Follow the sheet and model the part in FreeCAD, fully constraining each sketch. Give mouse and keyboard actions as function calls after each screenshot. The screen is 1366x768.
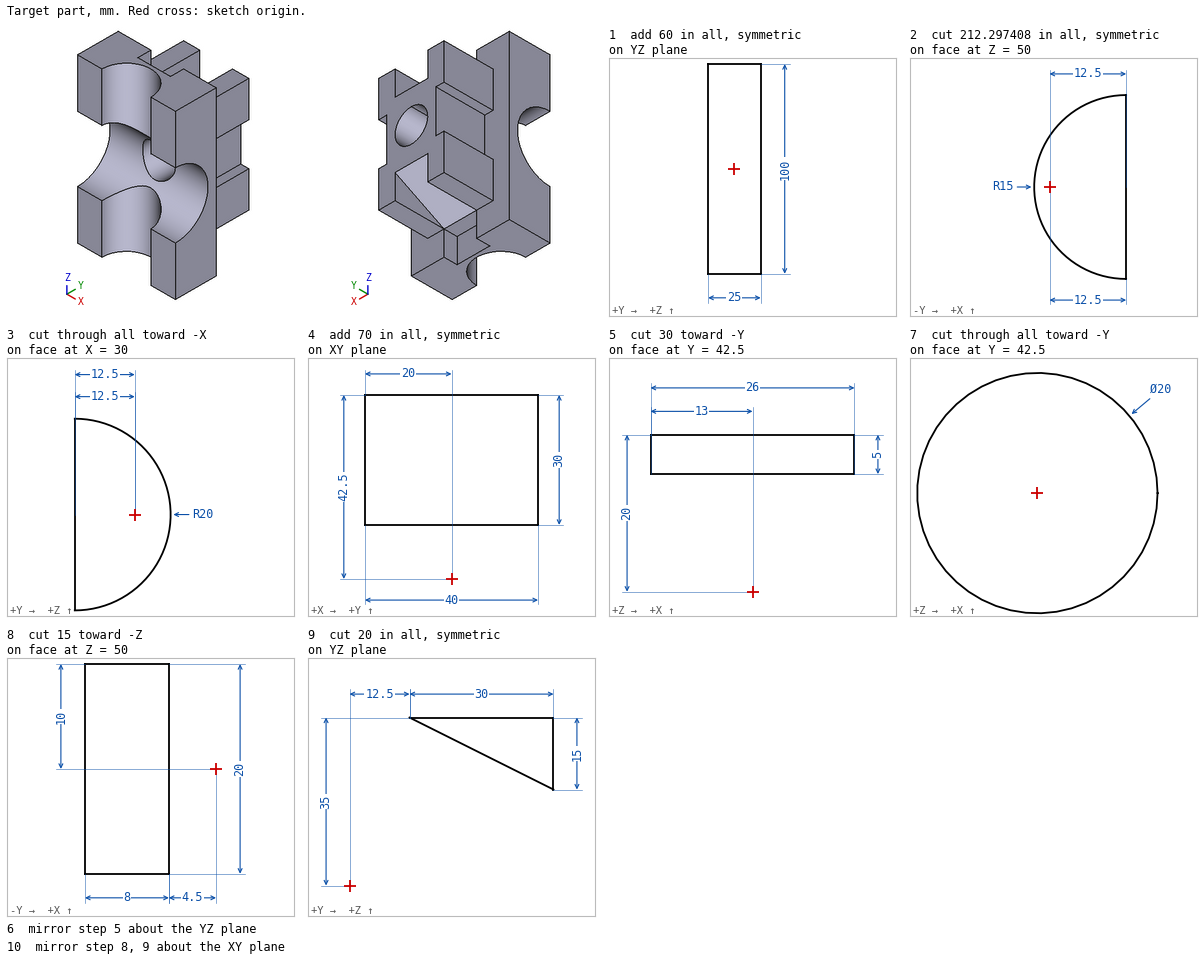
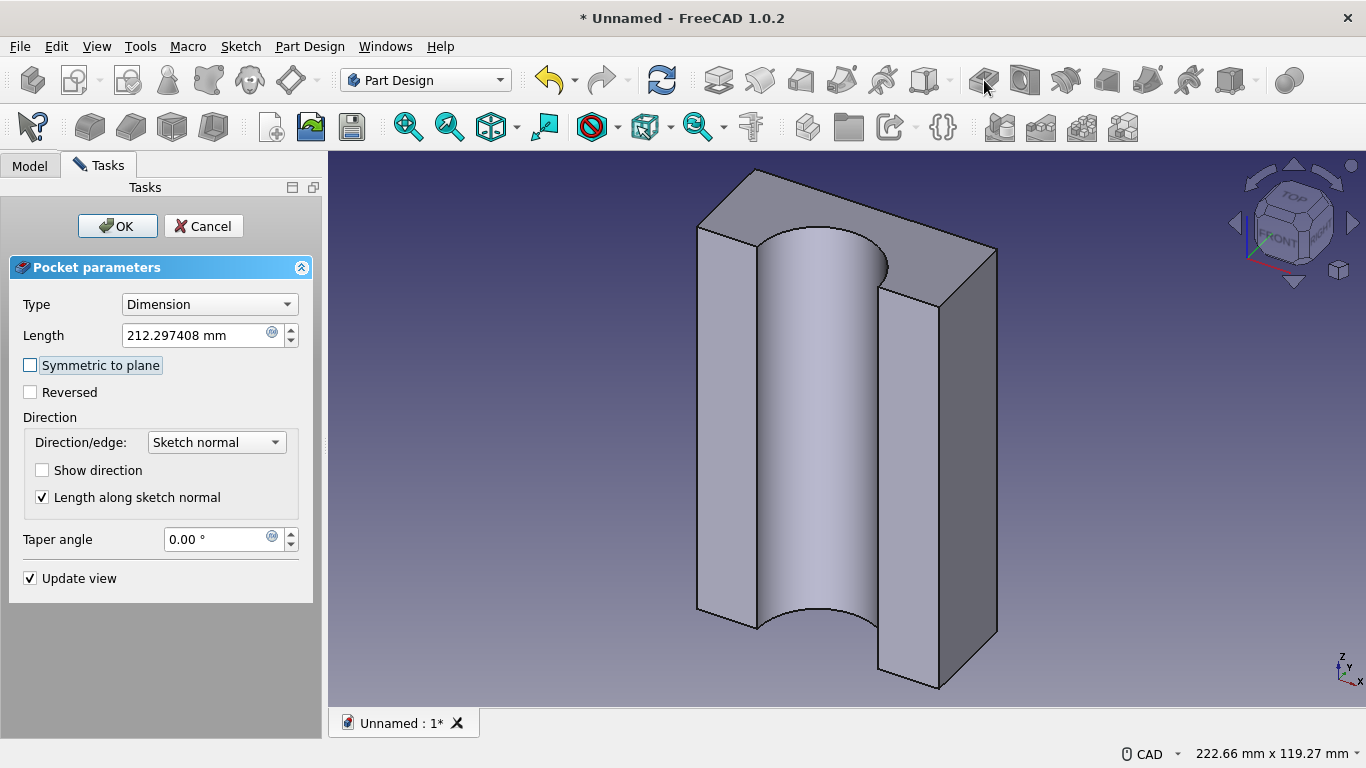
click(31, 365)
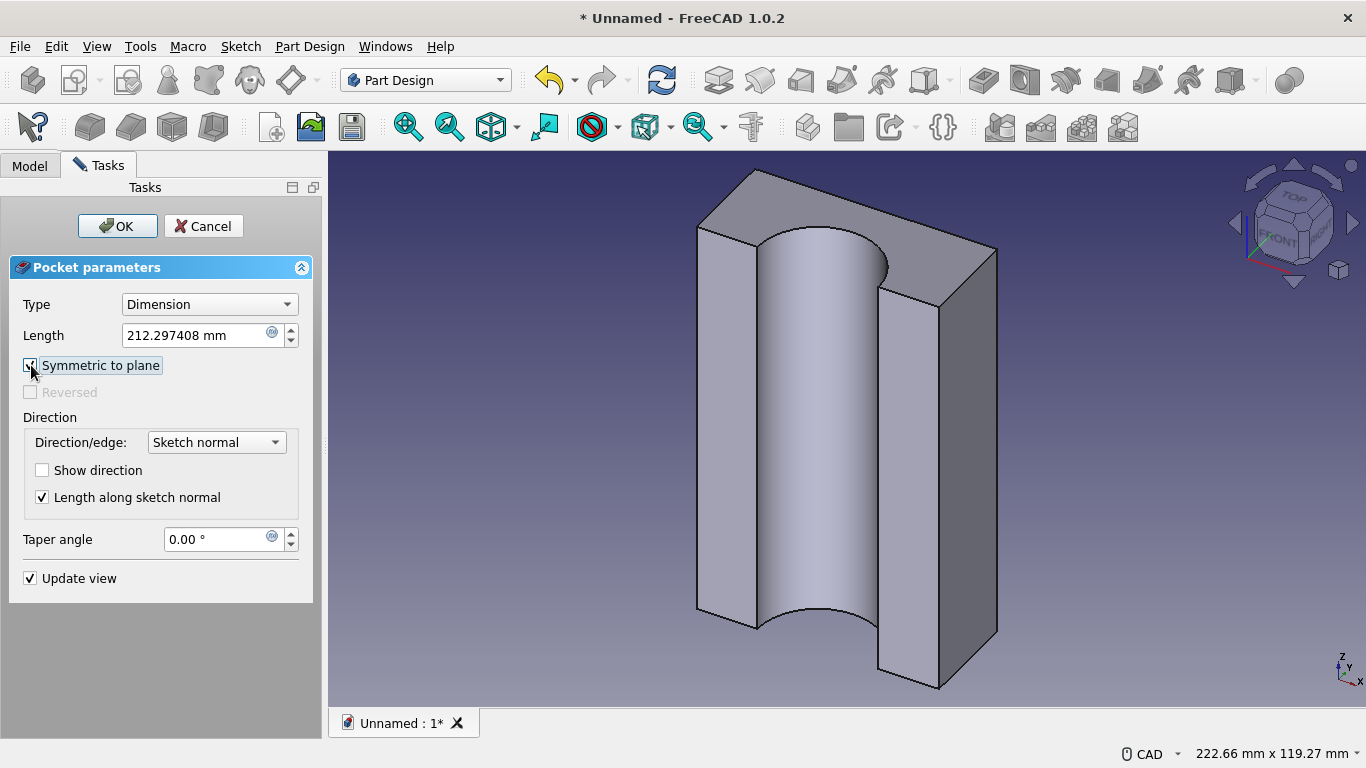
click(118, 226)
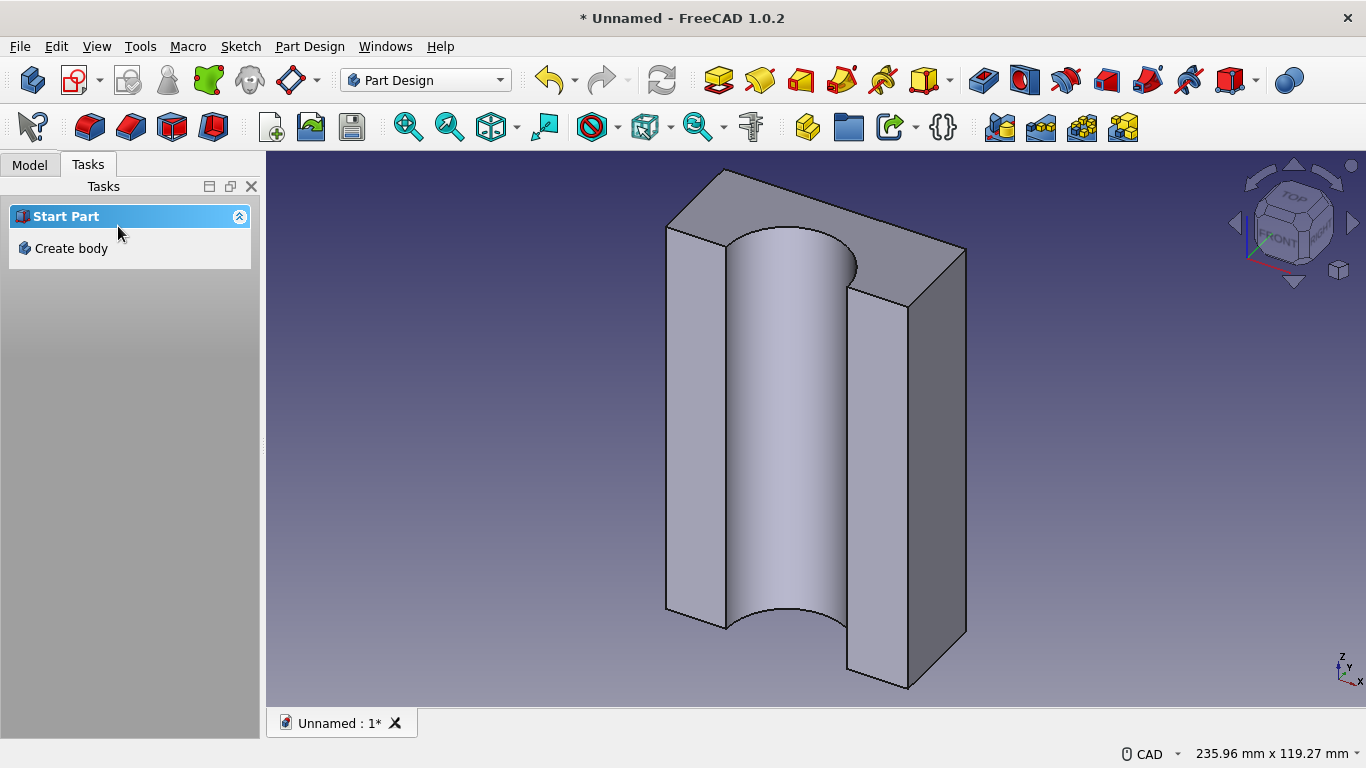
click(937, 577)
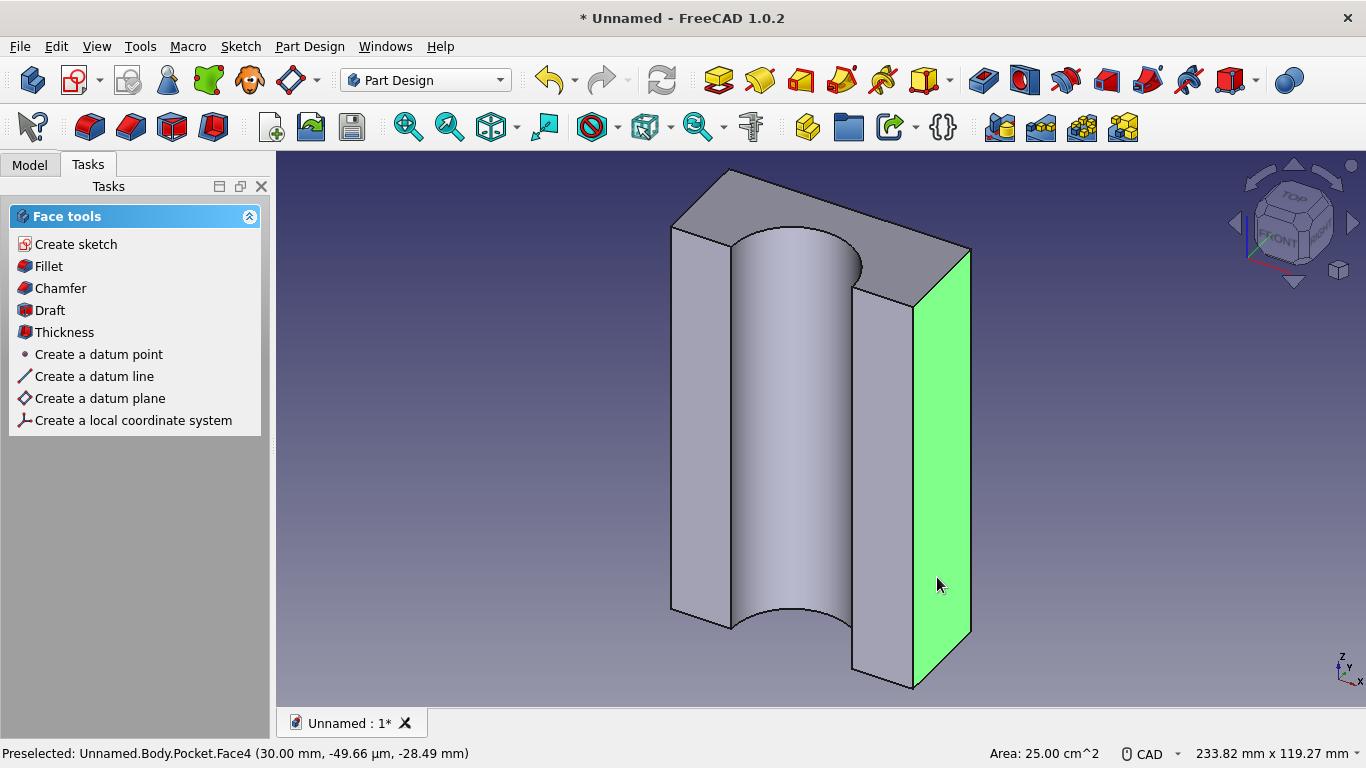
click(74, 80)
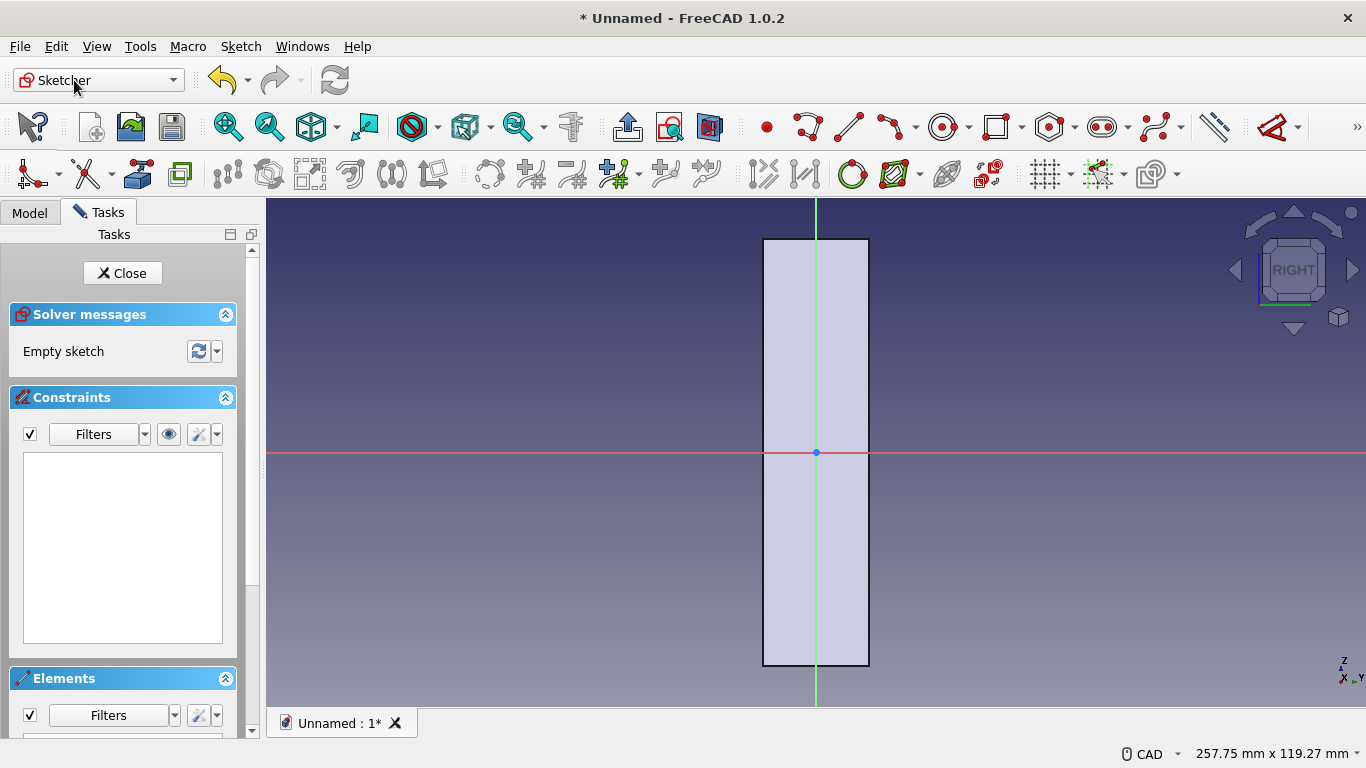
scroll(876, 452, up, 3)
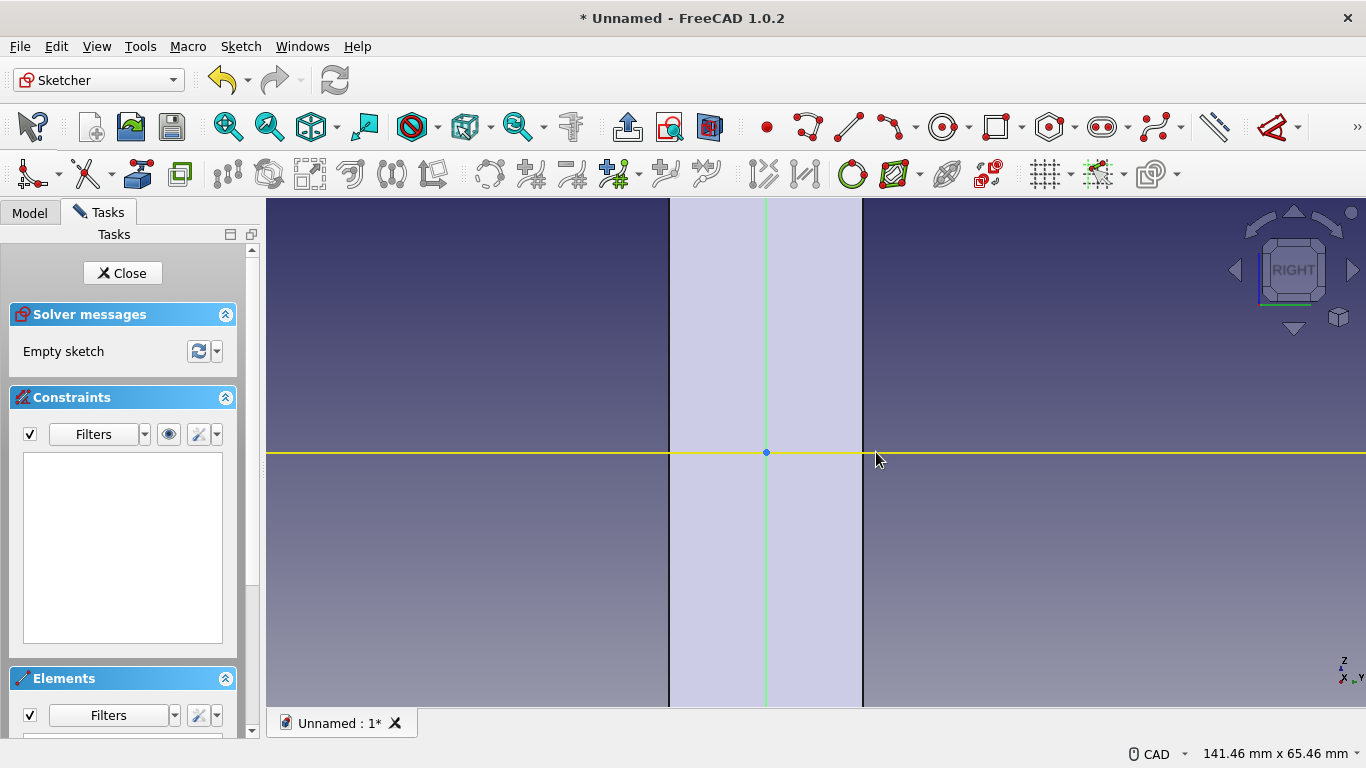
click(849, 128)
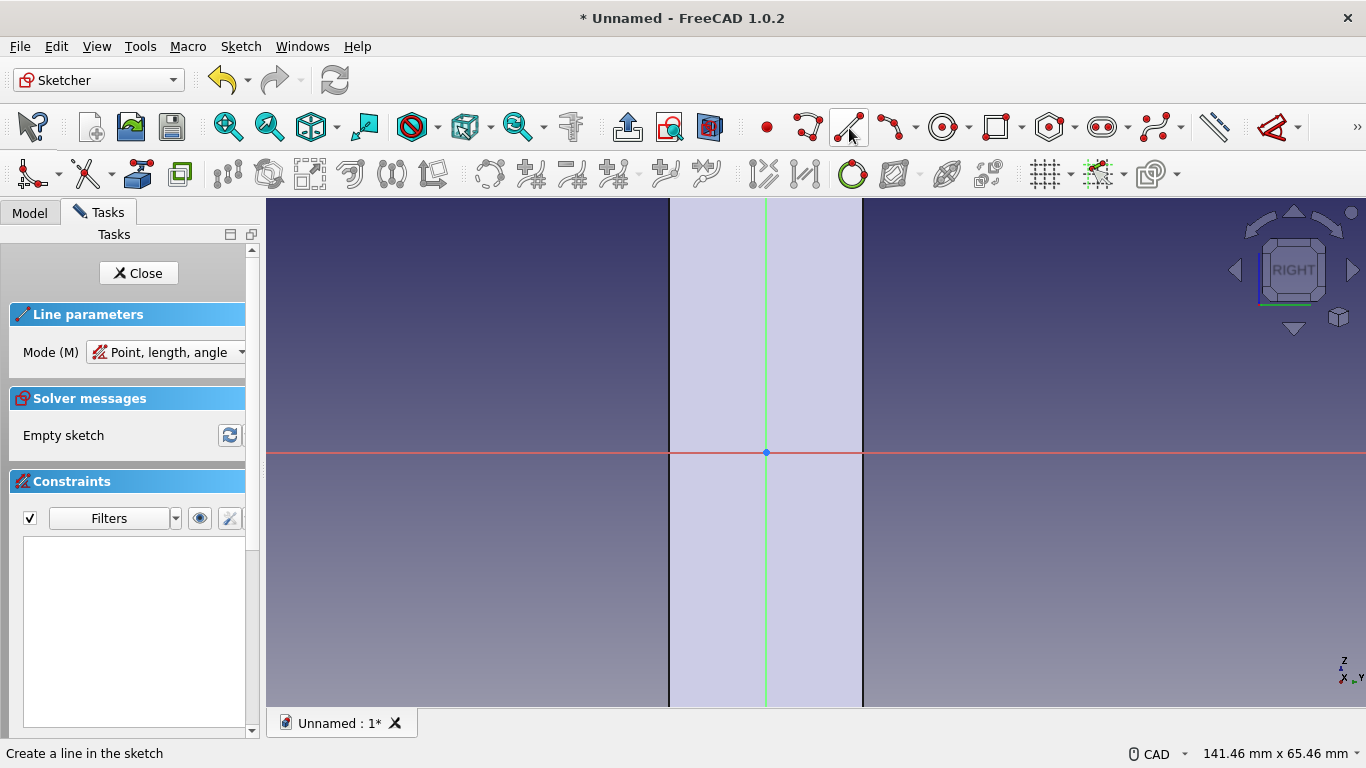
click(669, 297)
click(669, 608)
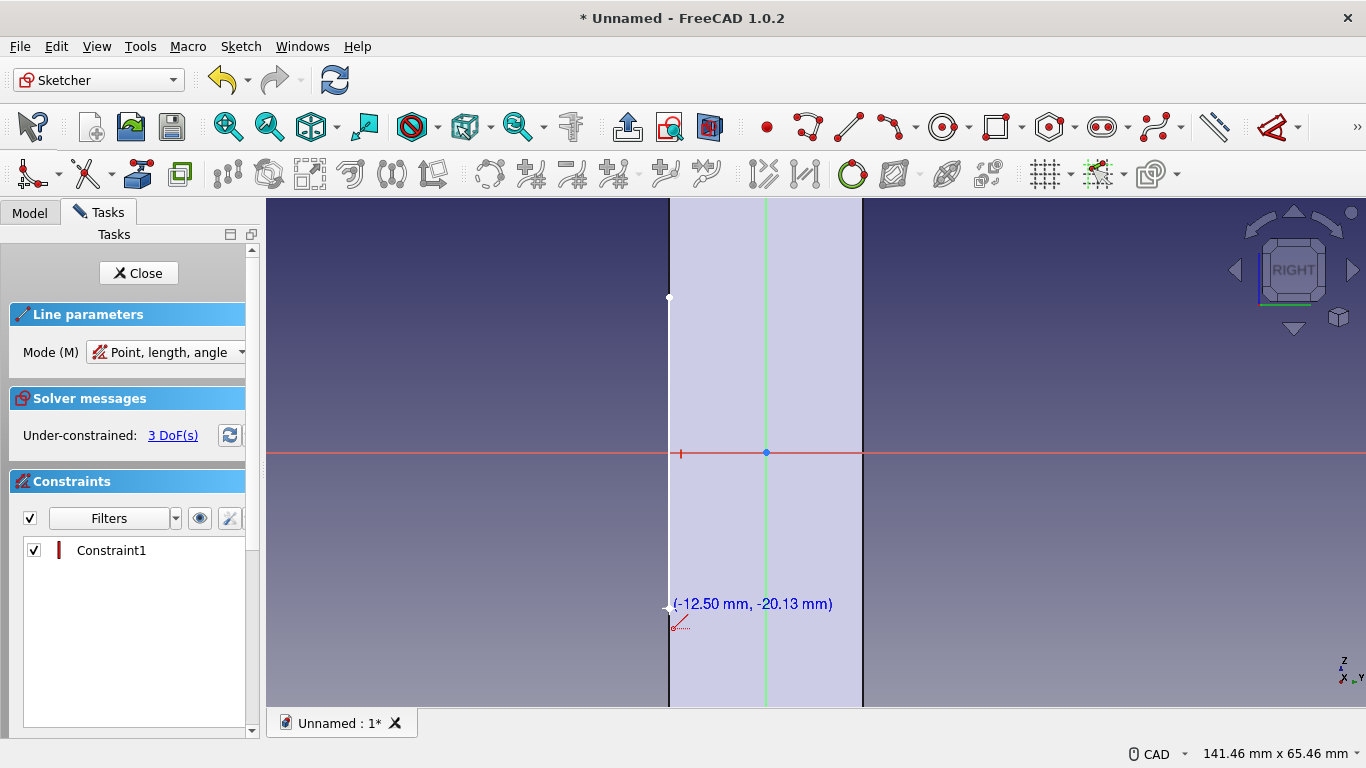
key(g)
key(3)
key(a)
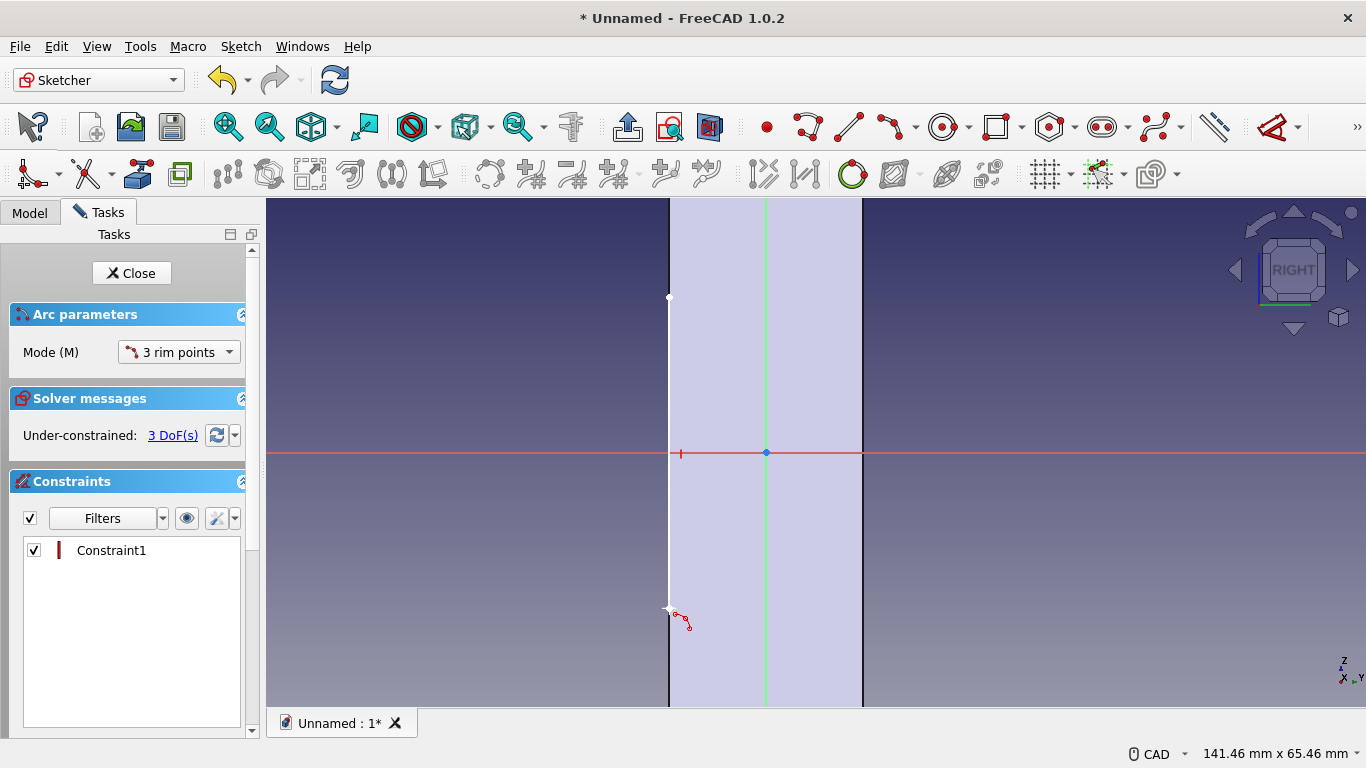
click(669, 609)
click(669, 298)
click(817, 501)
key(Escape)